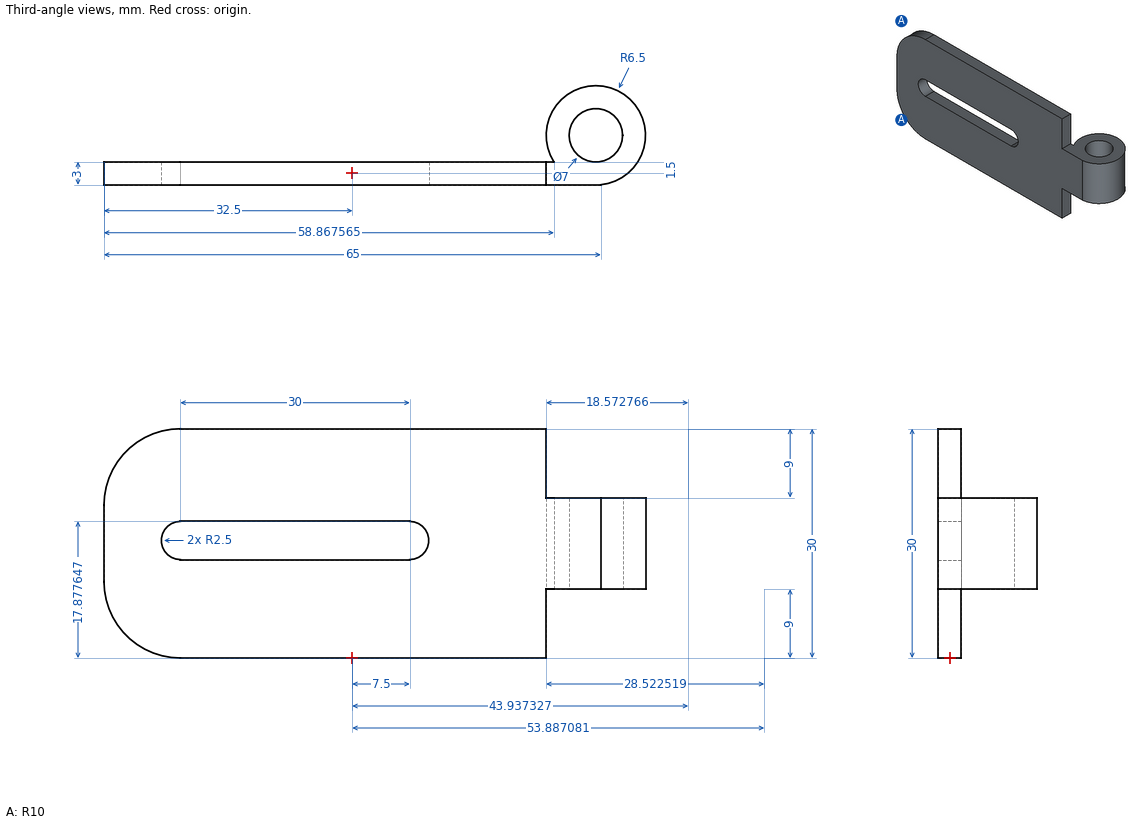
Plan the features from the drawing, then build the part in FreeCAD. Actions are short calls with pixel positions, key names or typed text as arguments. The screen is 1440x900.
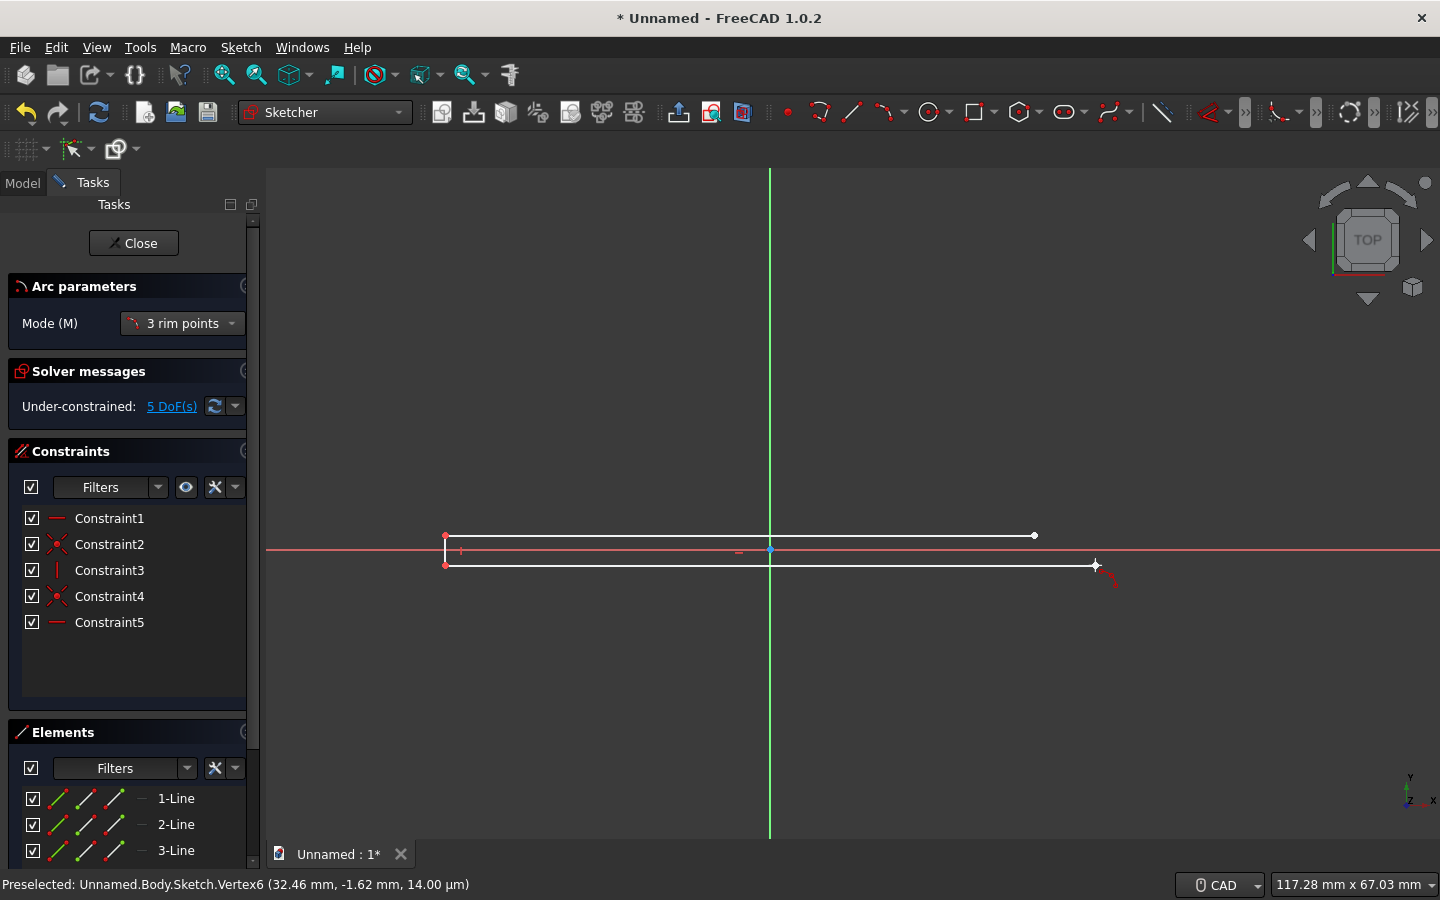
click(1095, 566)
click(1034, 536)
click(1118, 442)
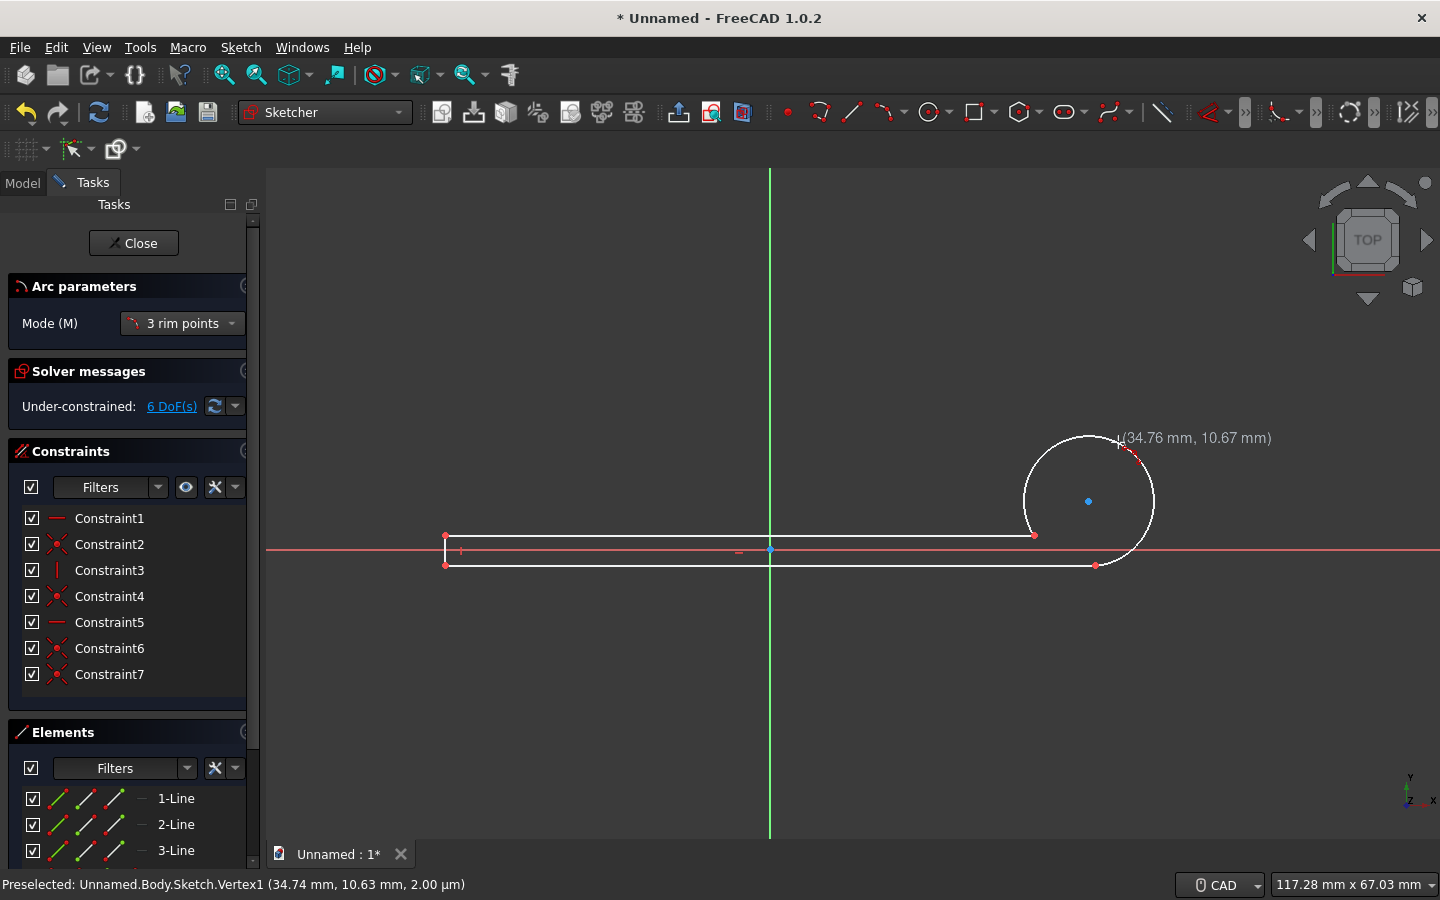
click(930, 112)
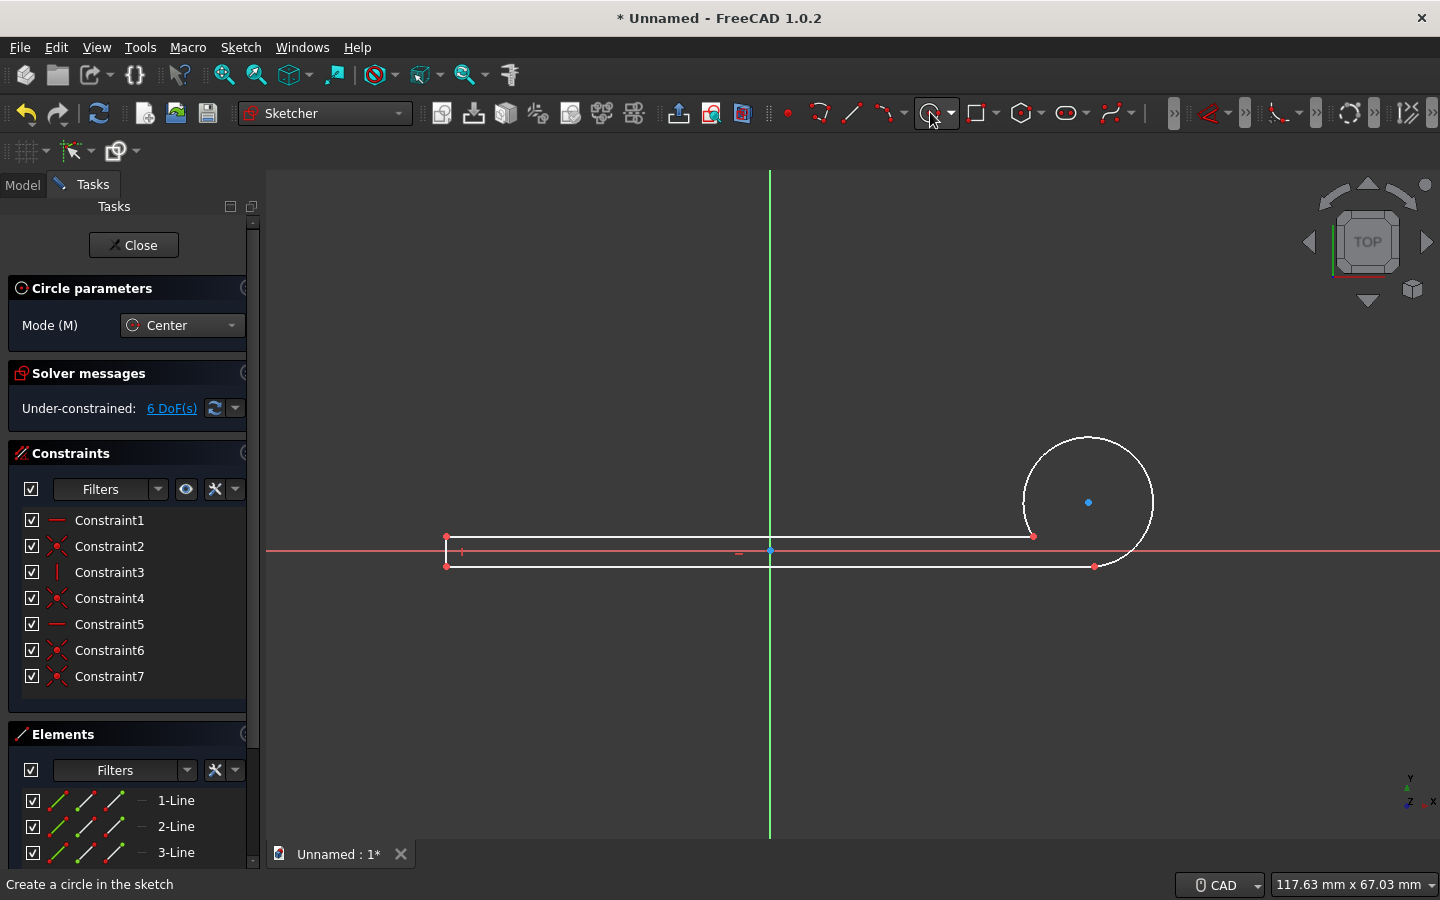
click(1088, 501)
move(1113, 476)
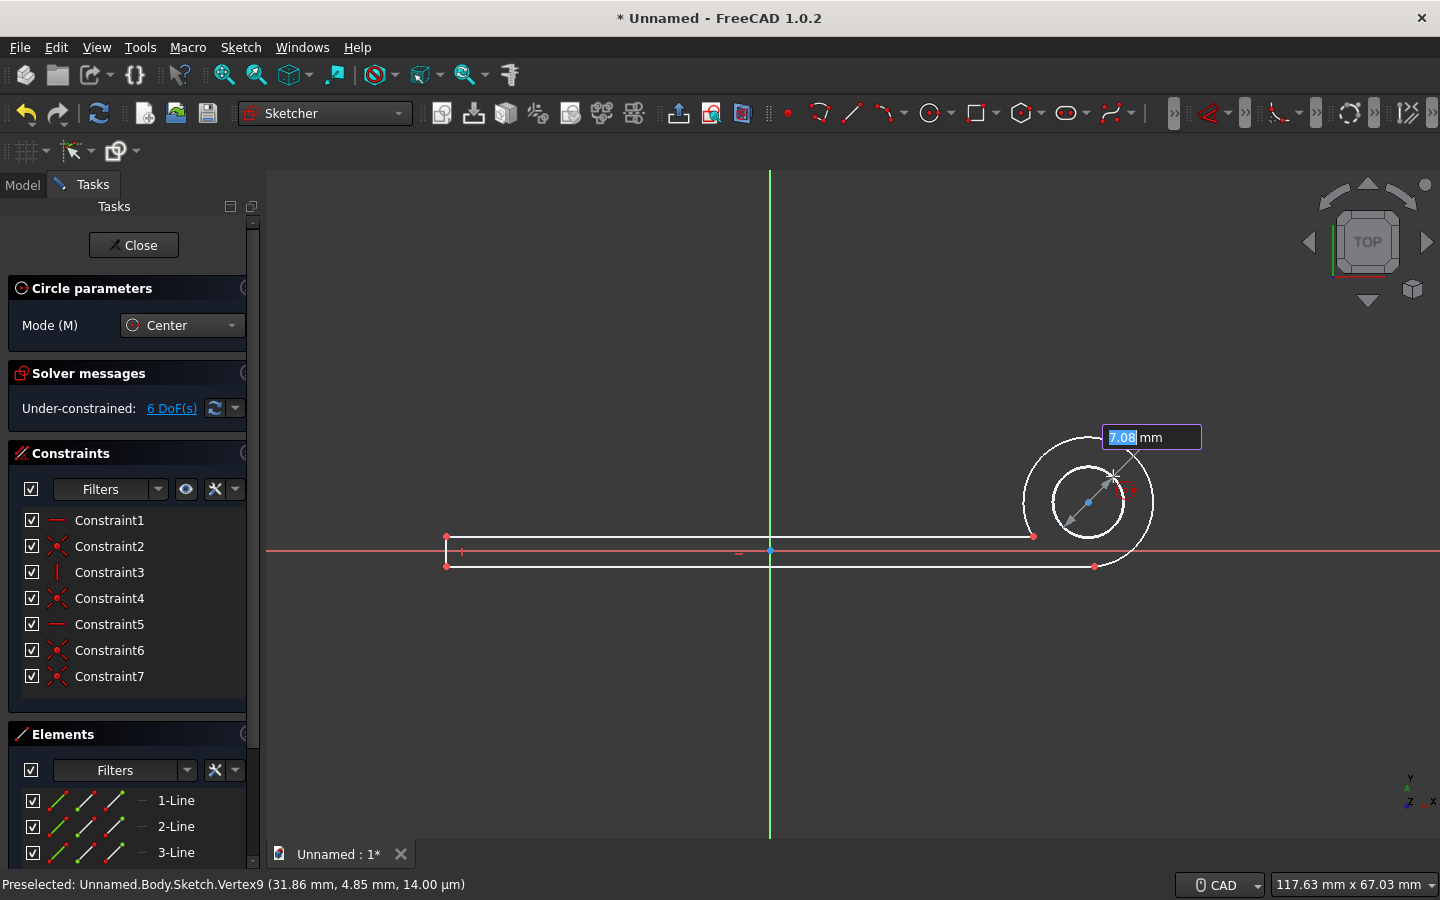
text(7)
key(Return)
key(Escape)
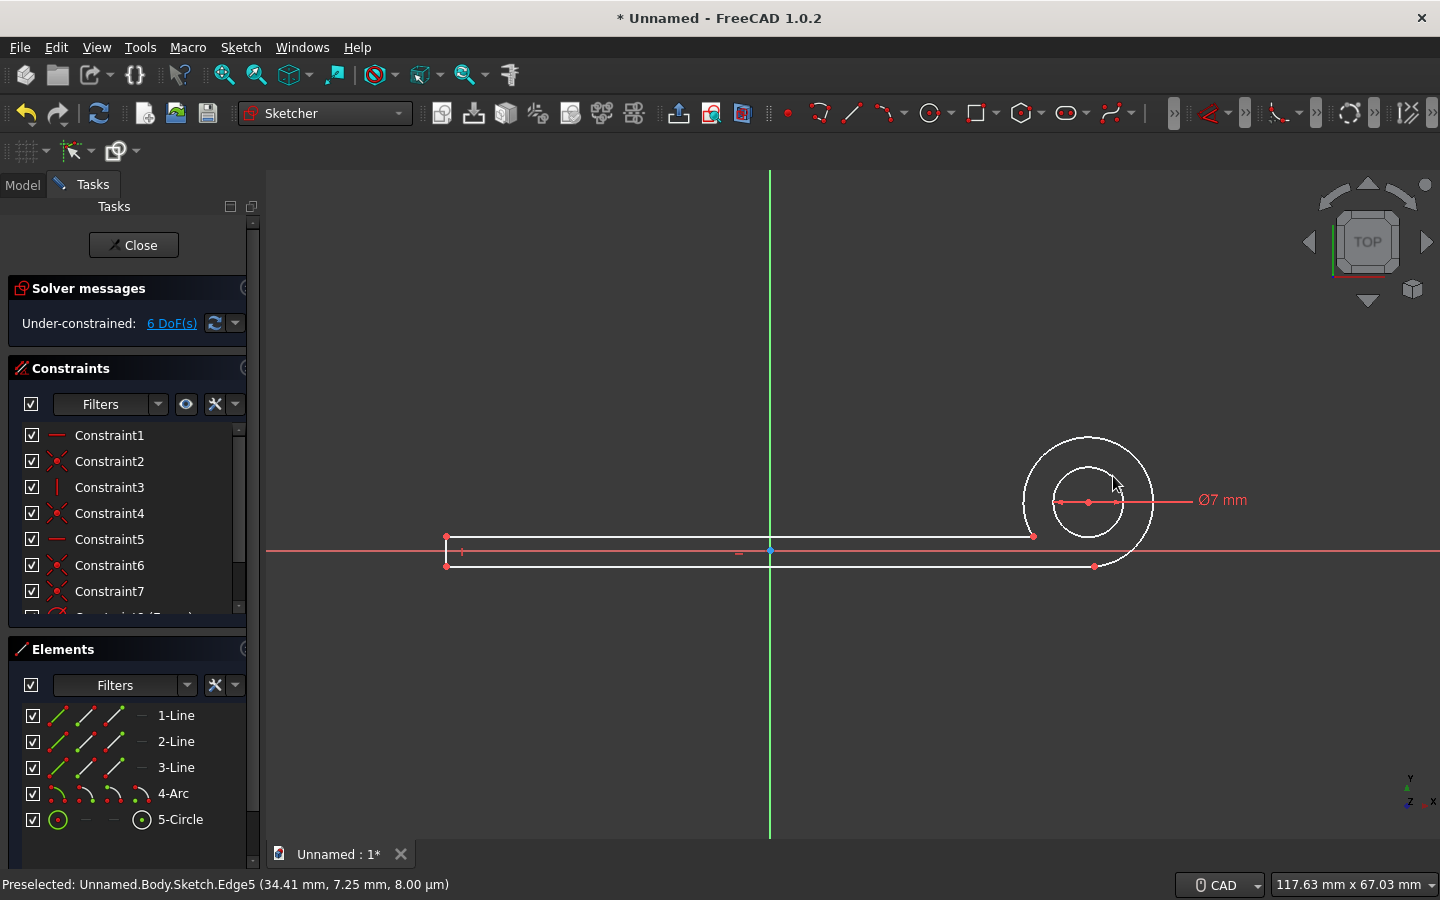
click(1208, 114)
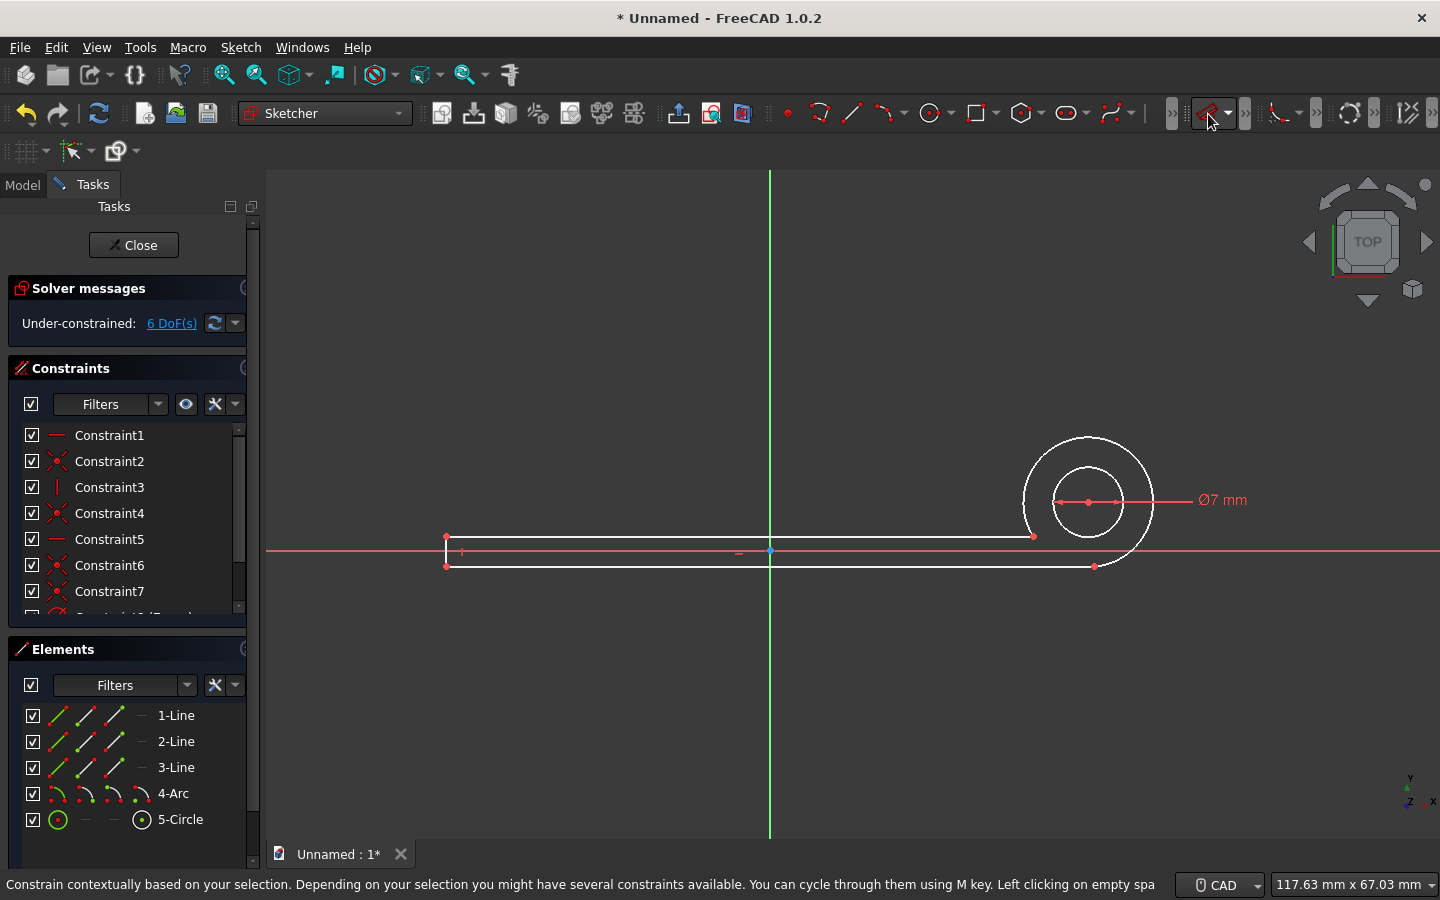
click(1153, 497)
click(1185, 494)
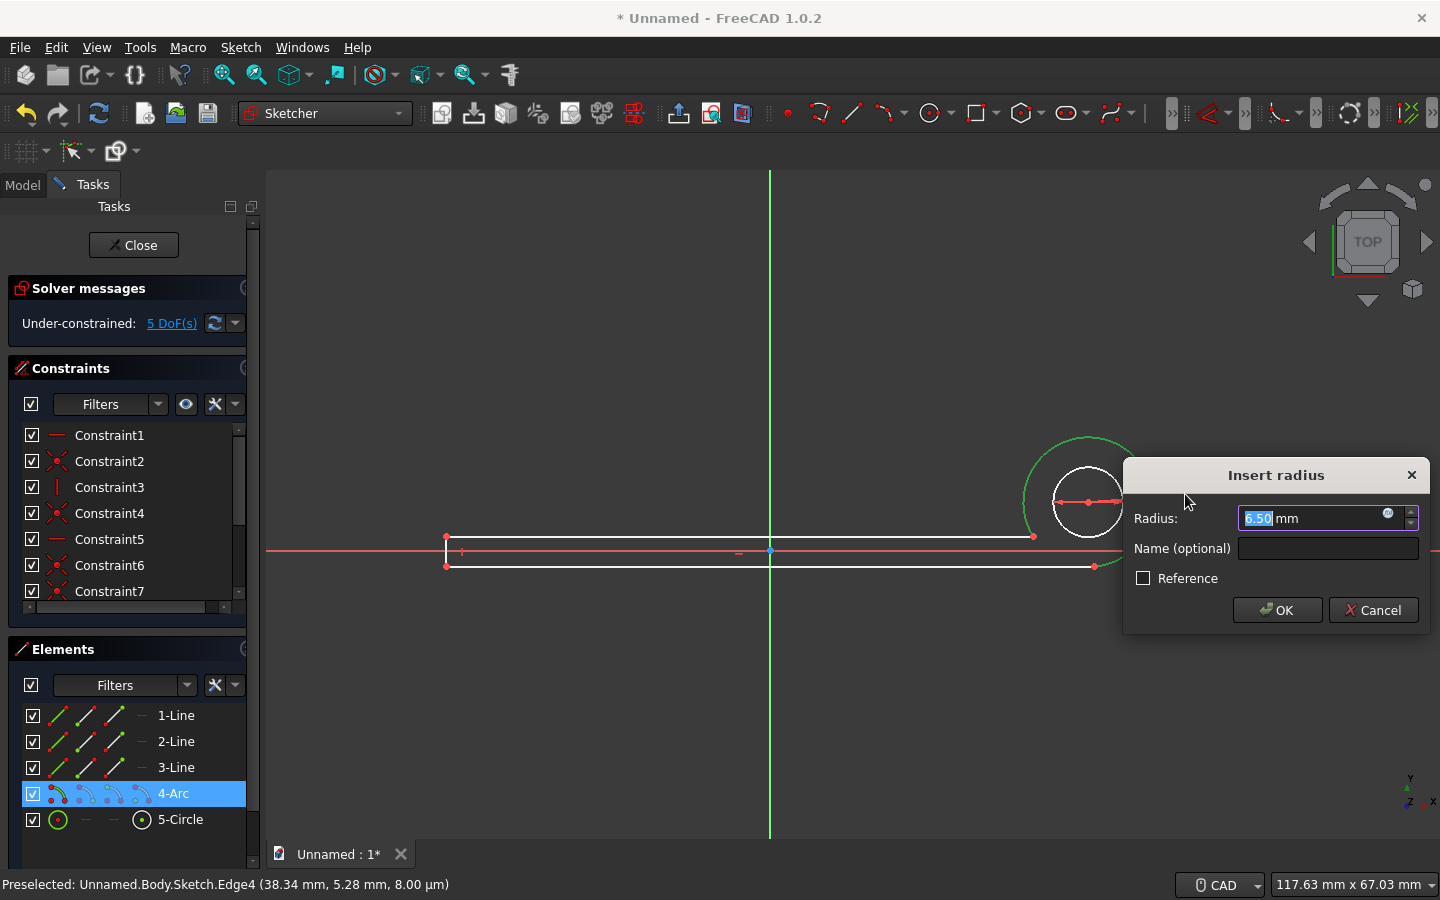
text(6.5)
key(Return)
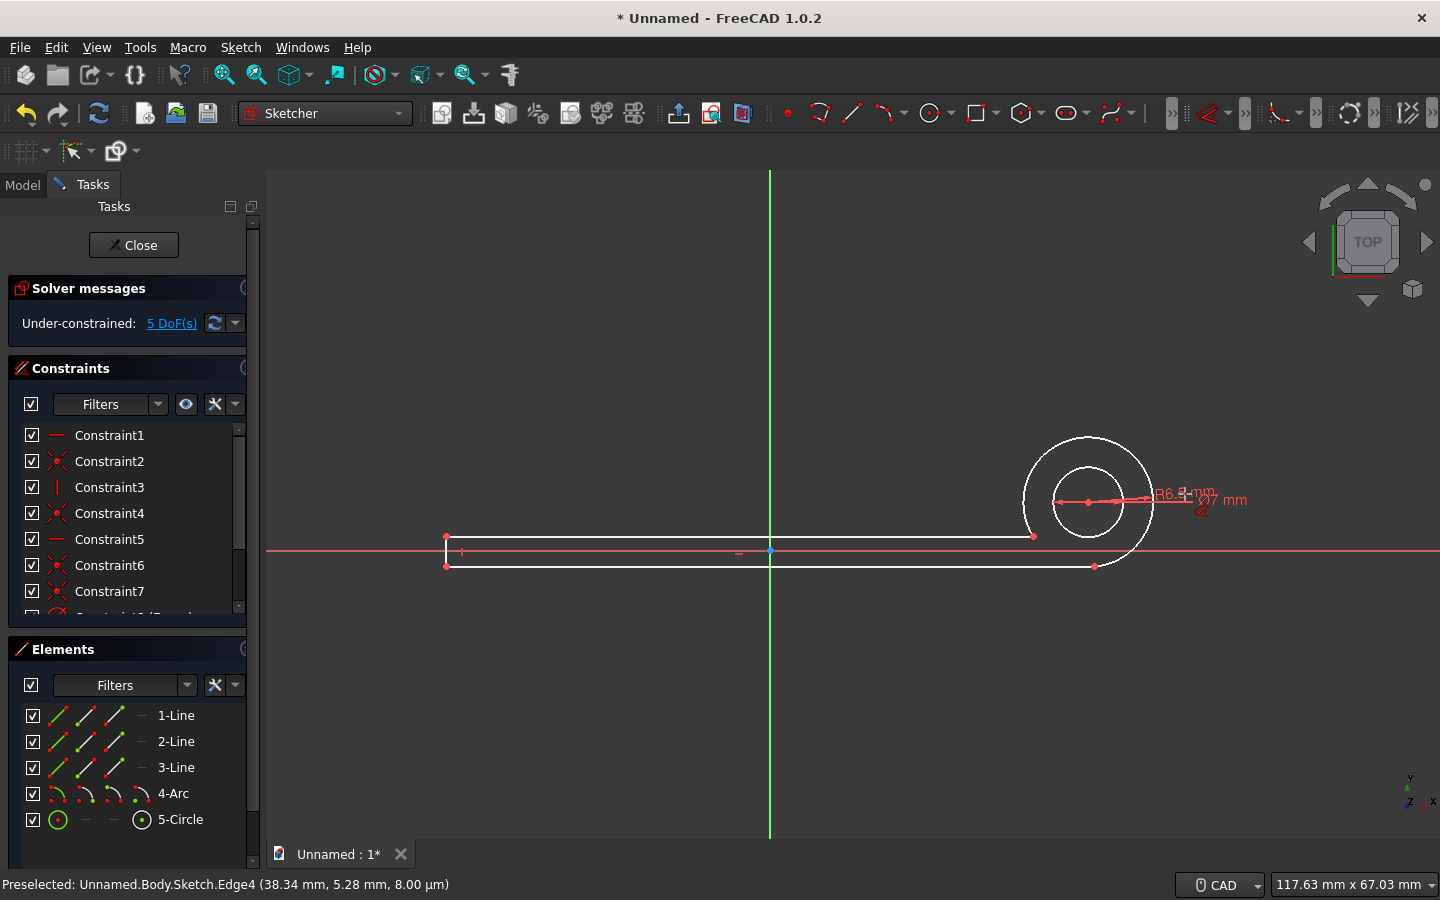
scroll(446, 549, up, 2)